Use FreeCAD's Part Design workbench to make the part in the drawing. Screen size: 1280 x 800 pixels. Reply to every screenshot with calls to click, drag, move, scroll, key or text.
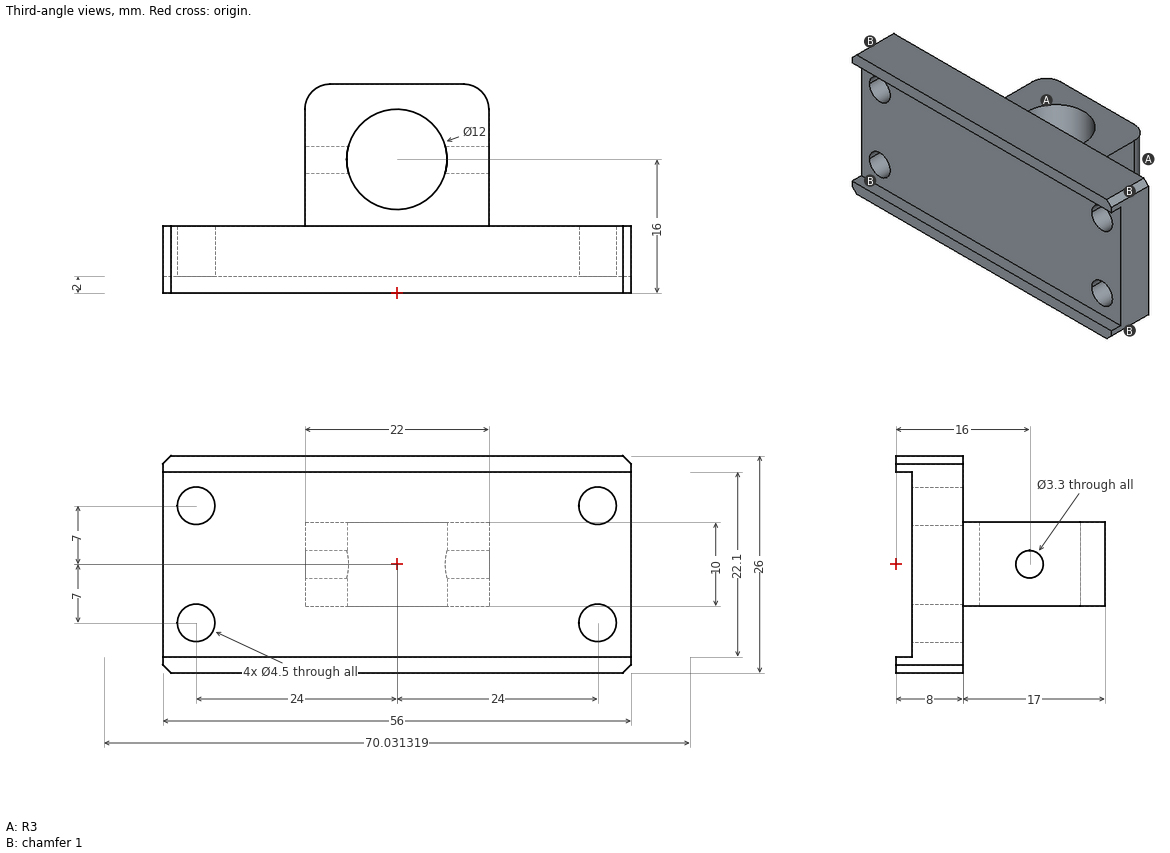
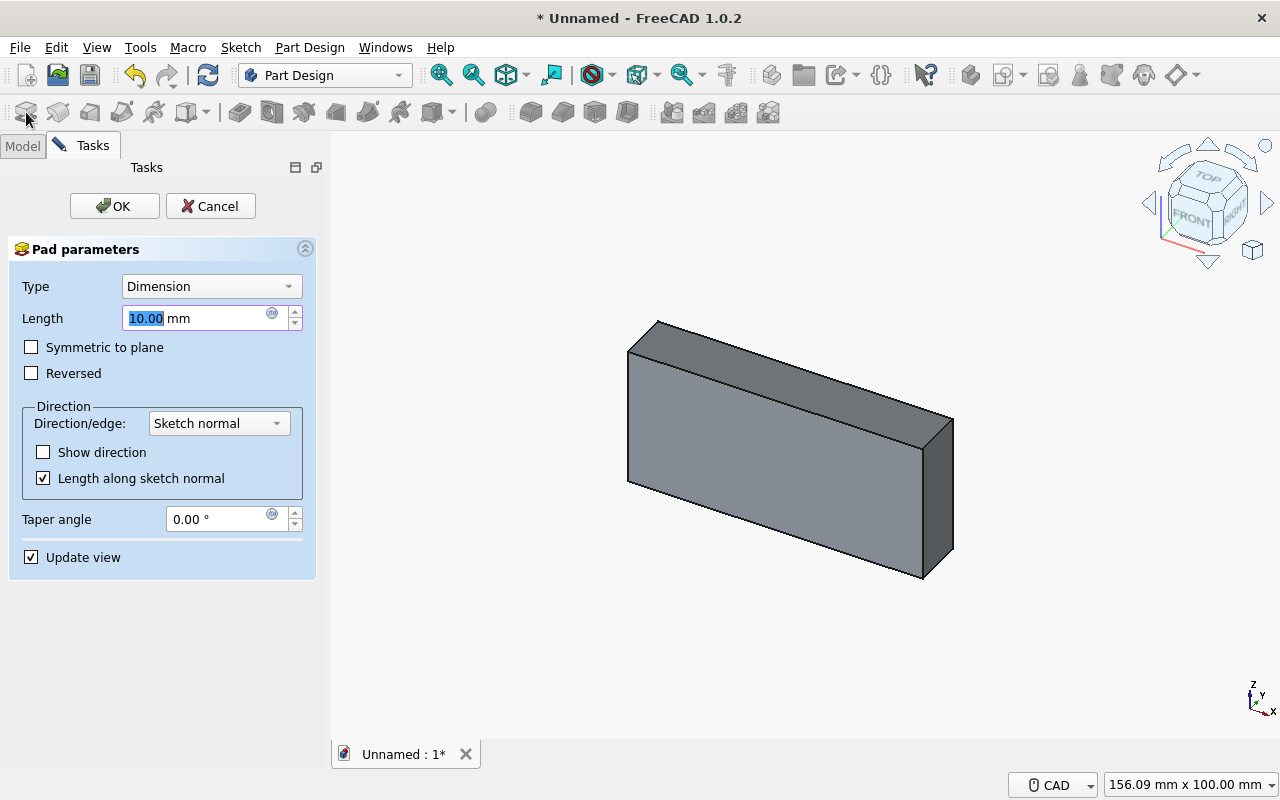
text(8)
key(Tab)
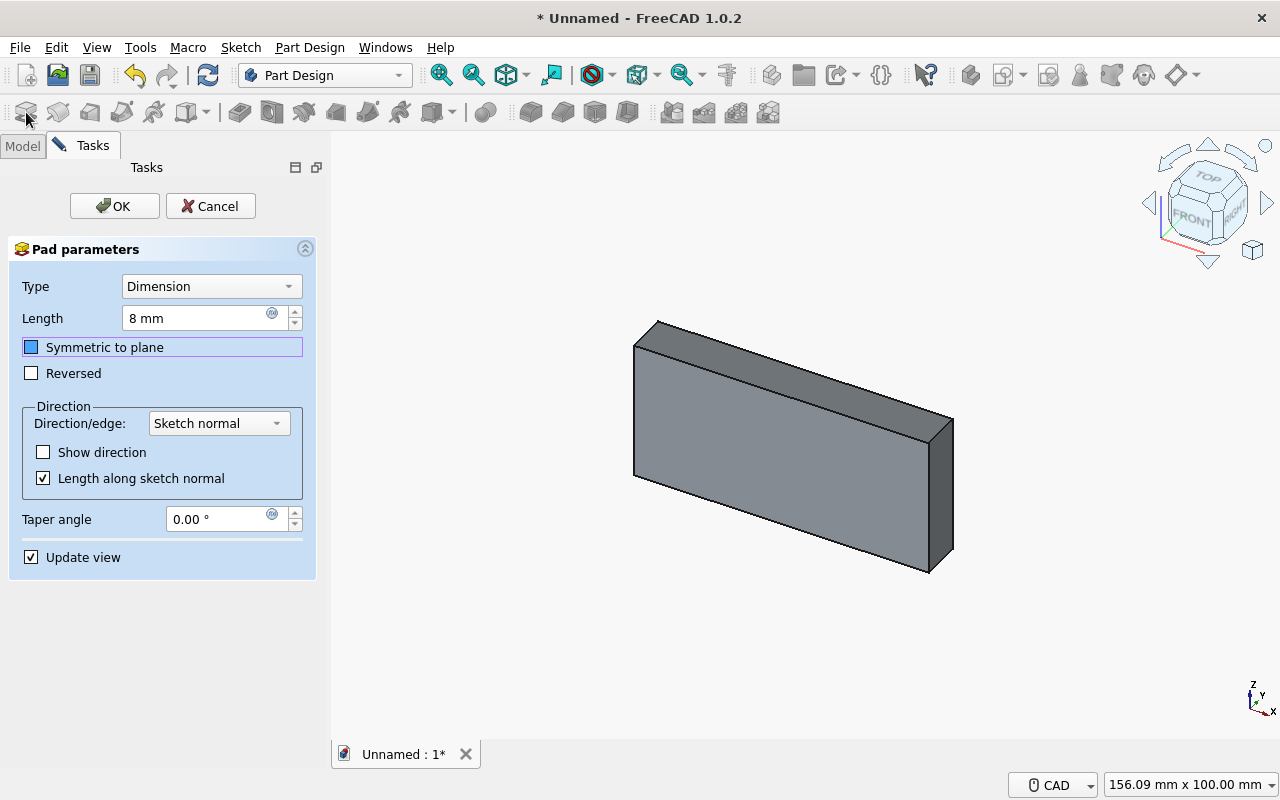
click(30, 373)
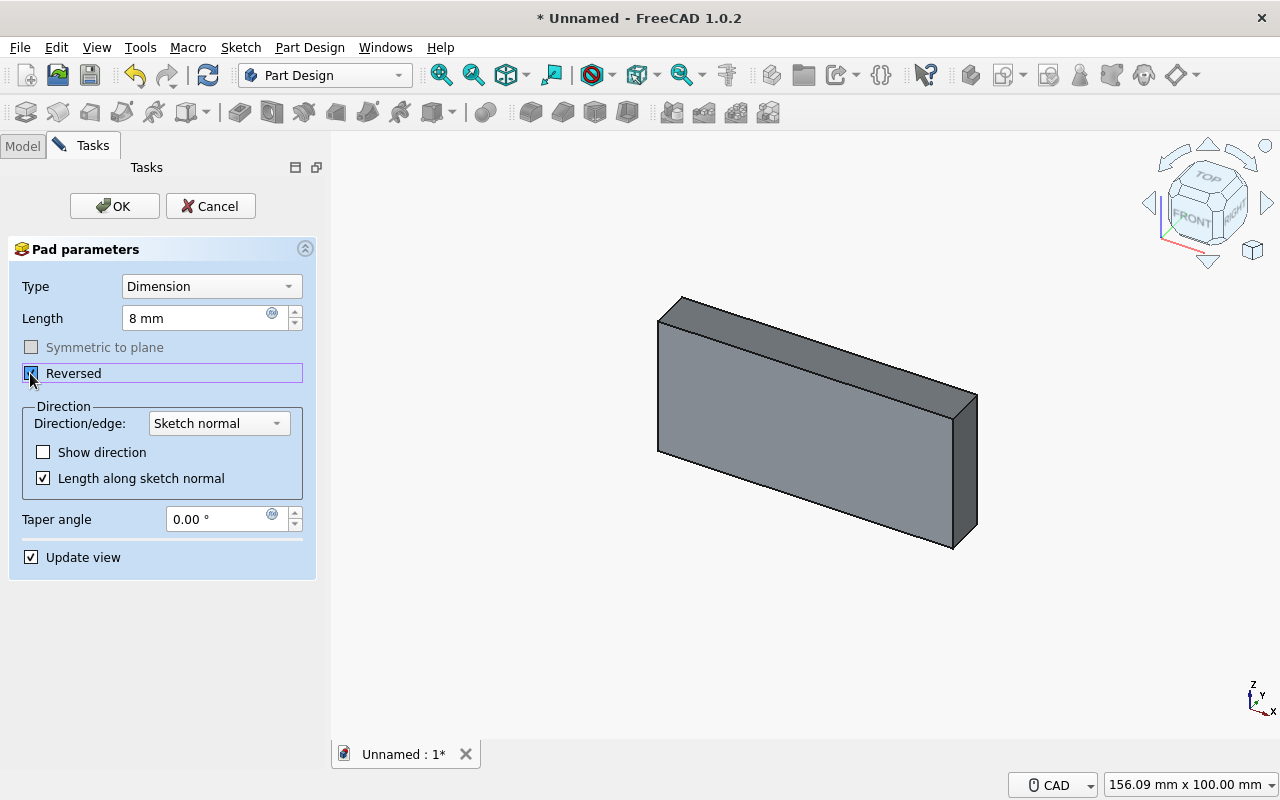
click(115, 206)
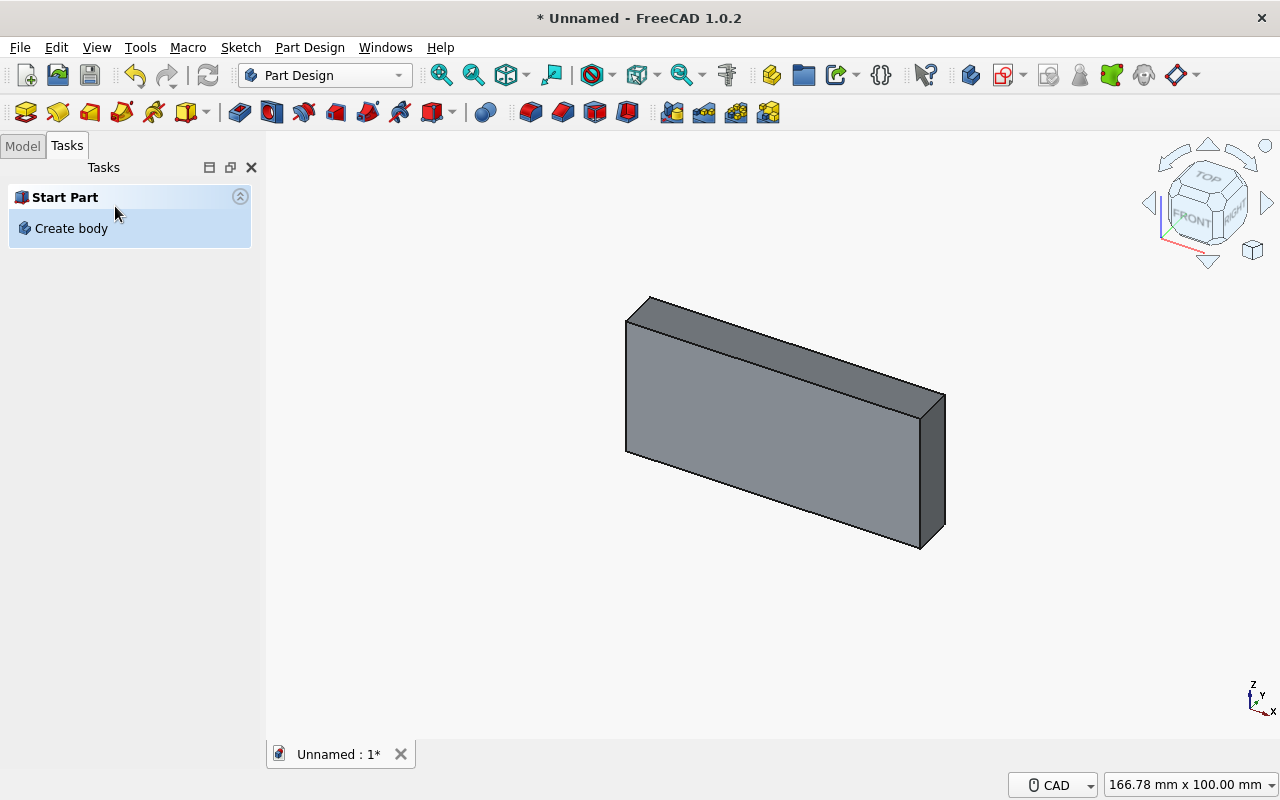
click(442, 76)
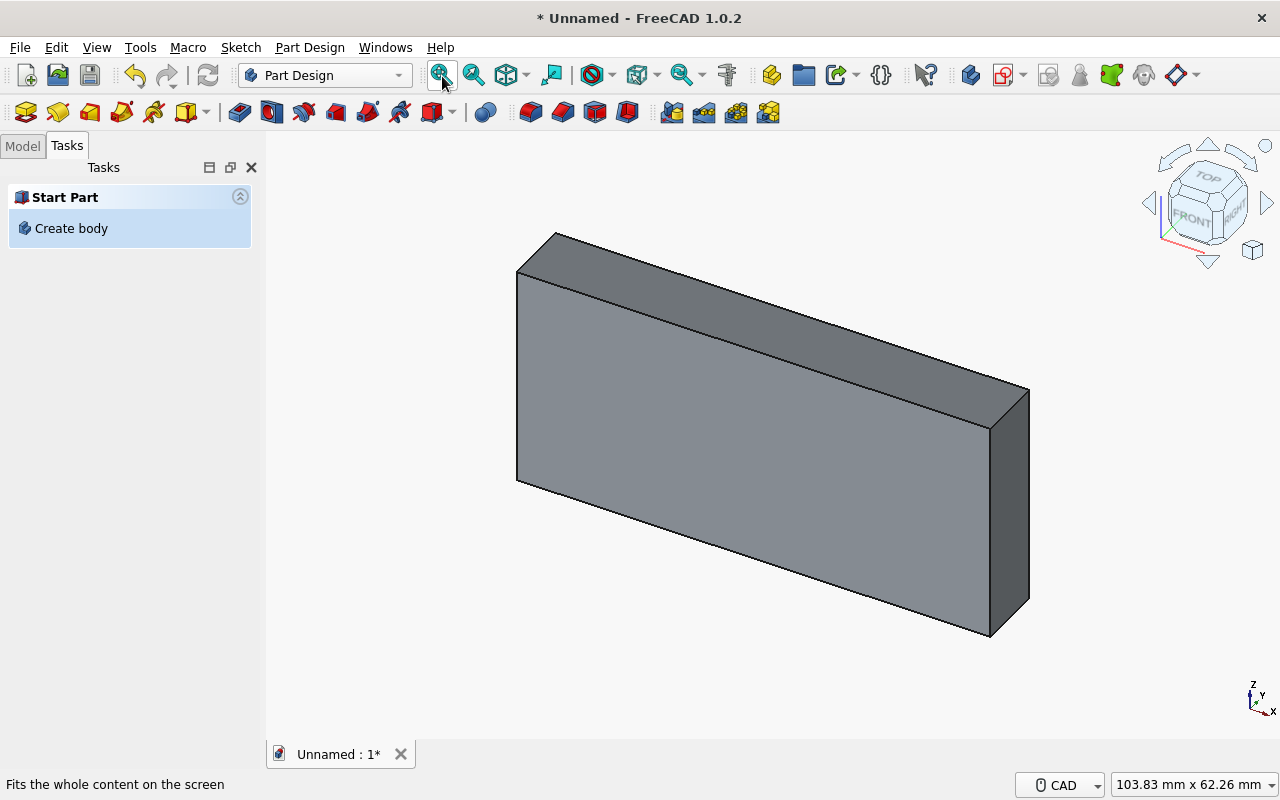
click(821, 476)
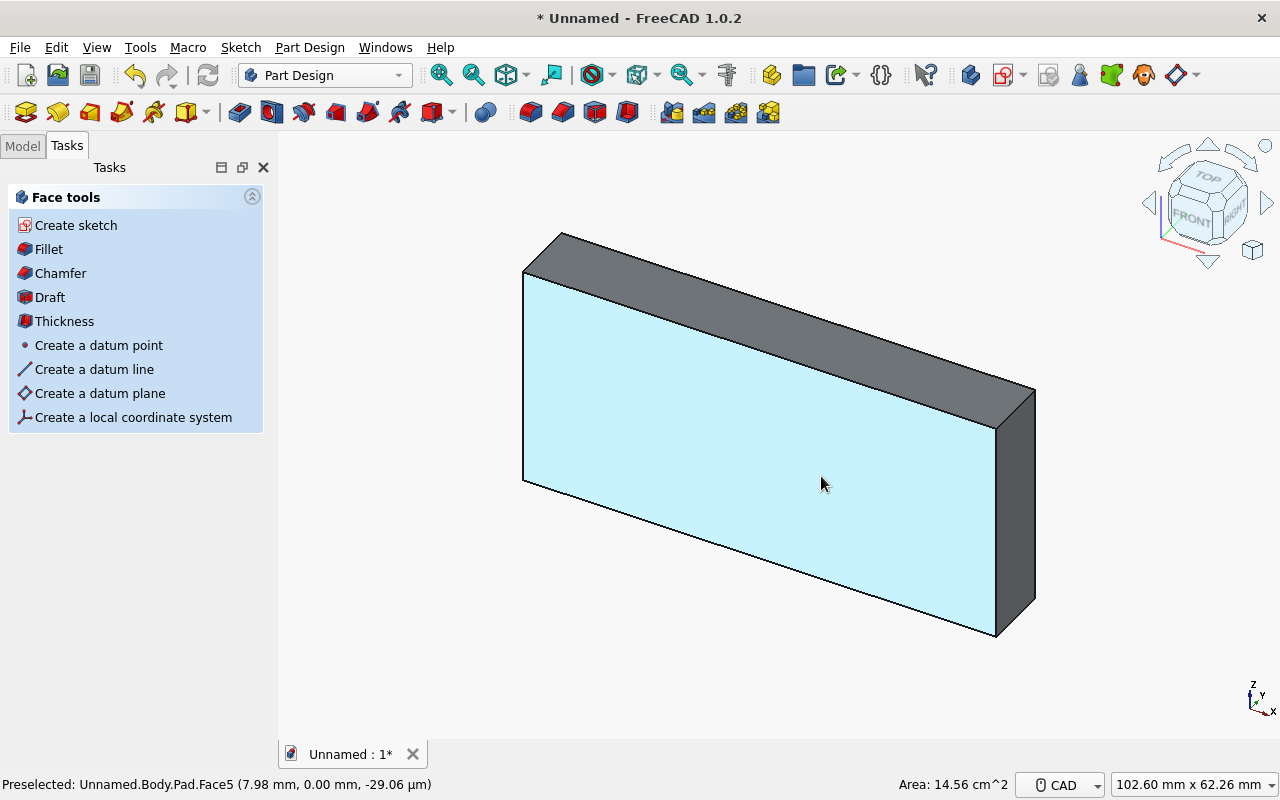
click(1004, 76)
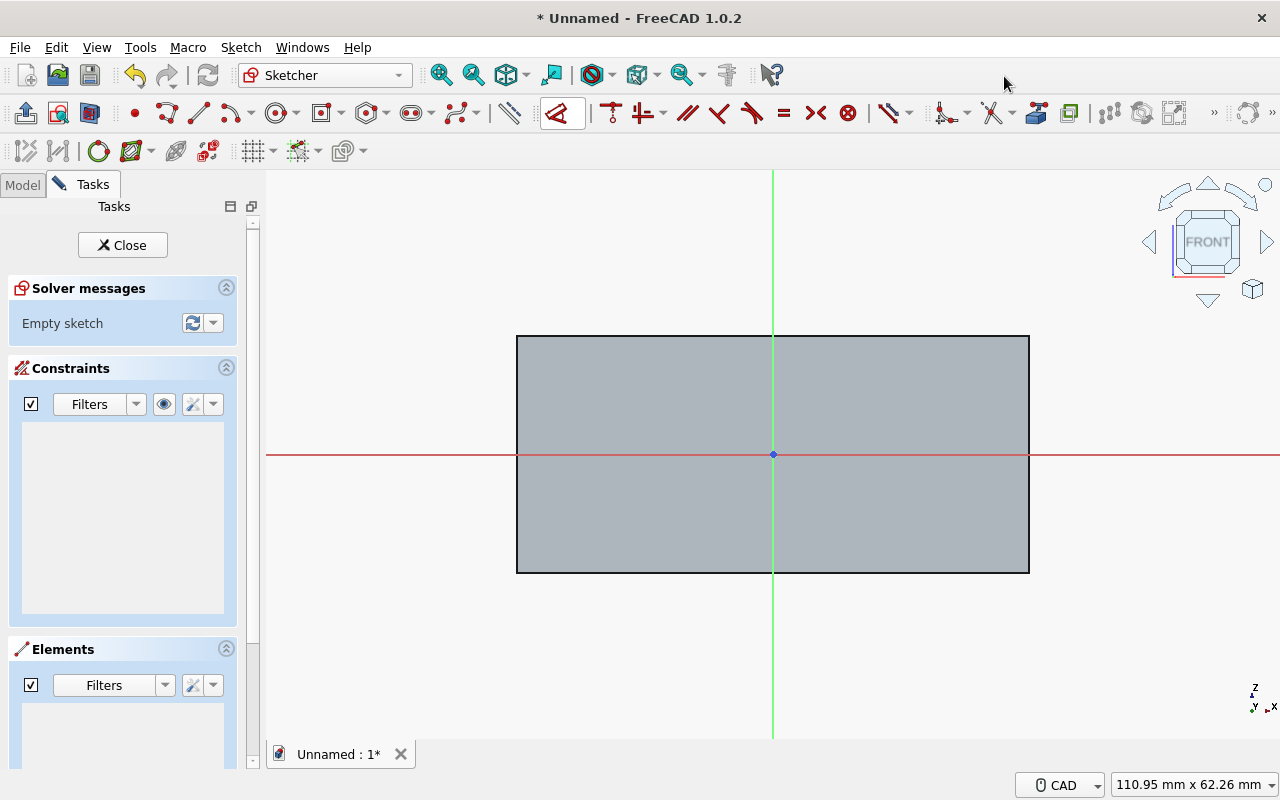
scroll(395, 454, down, 1)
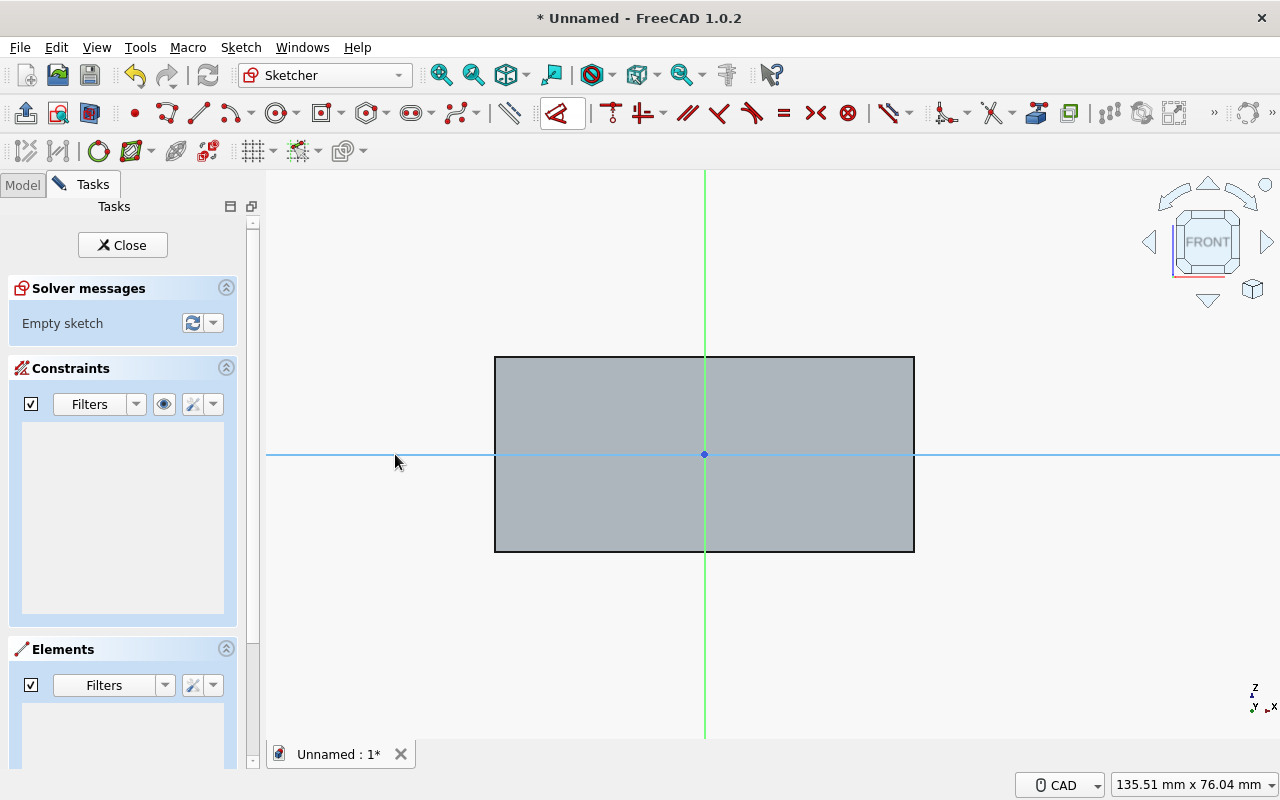
click(322, 114)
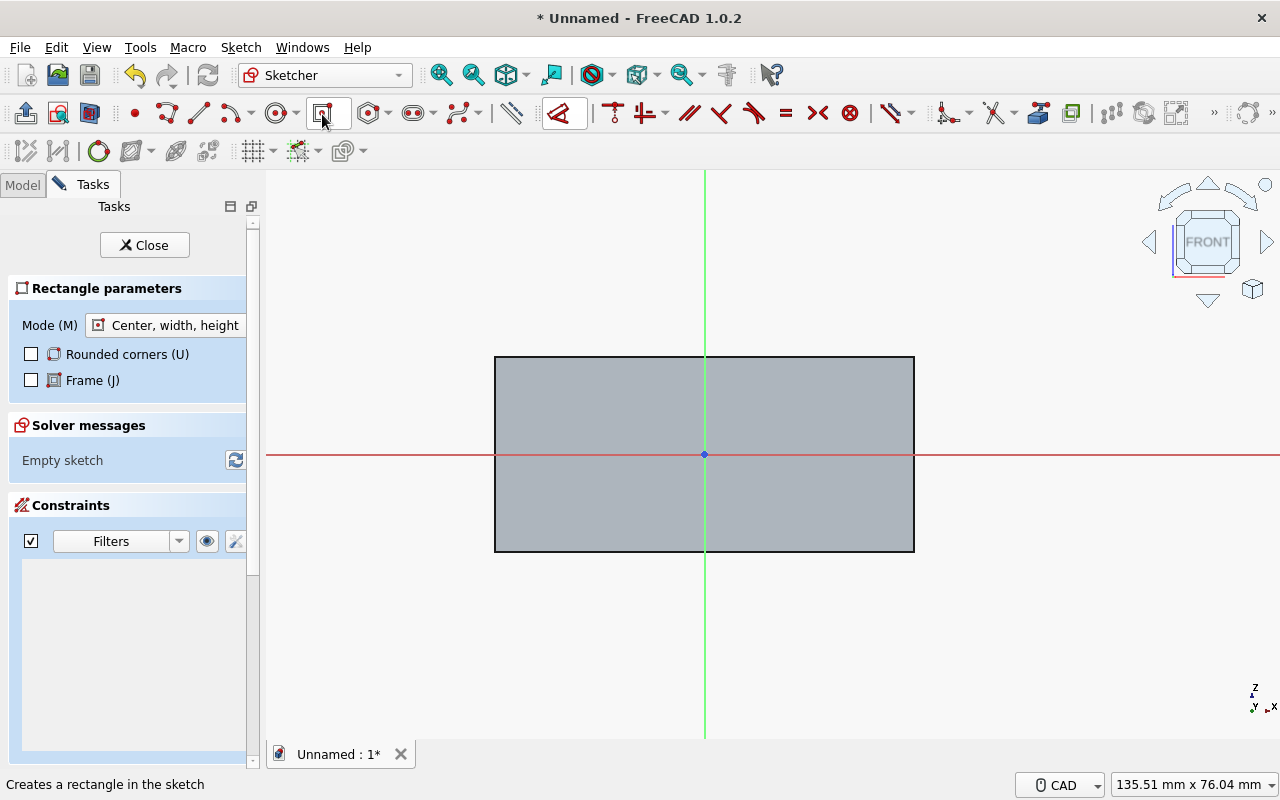
click(705, 455)
move(967, 372)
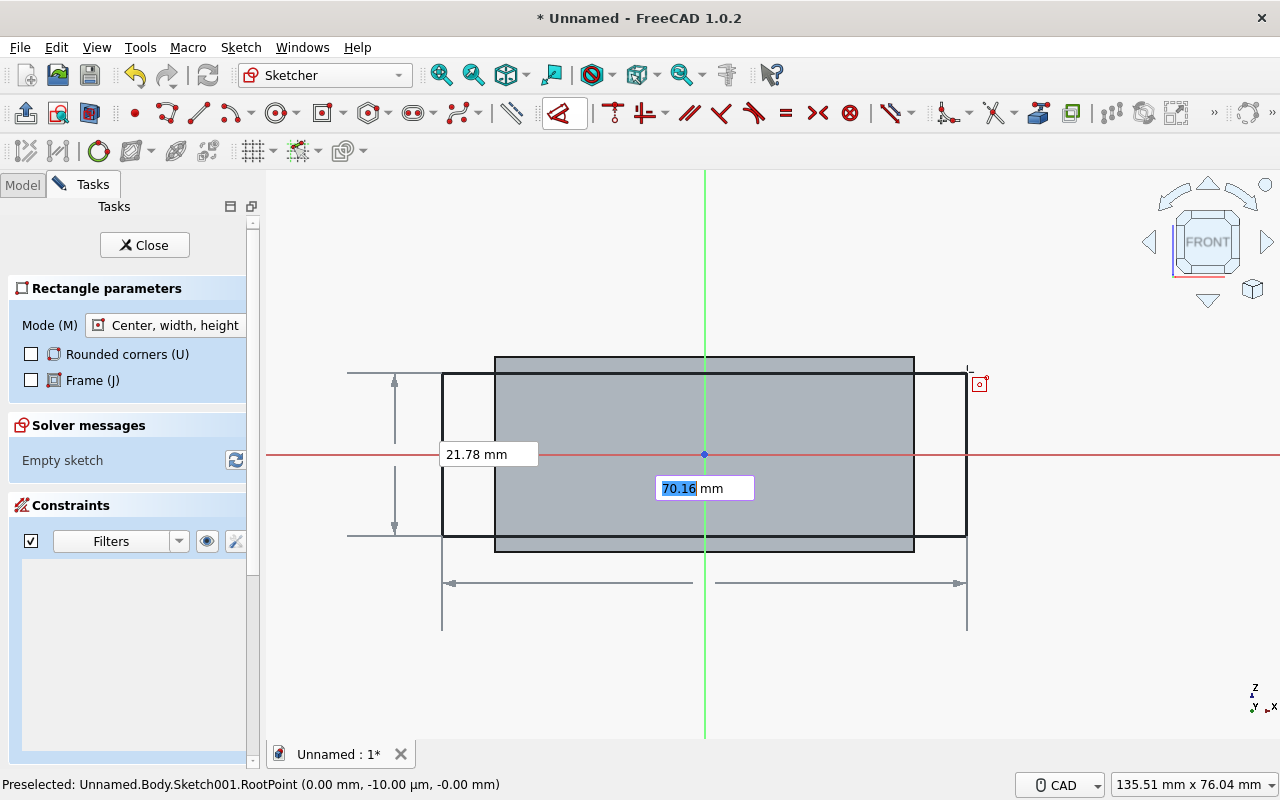
text(70.031319)
key(Tab)
text(22.1)
key(Return)
key(Escape)